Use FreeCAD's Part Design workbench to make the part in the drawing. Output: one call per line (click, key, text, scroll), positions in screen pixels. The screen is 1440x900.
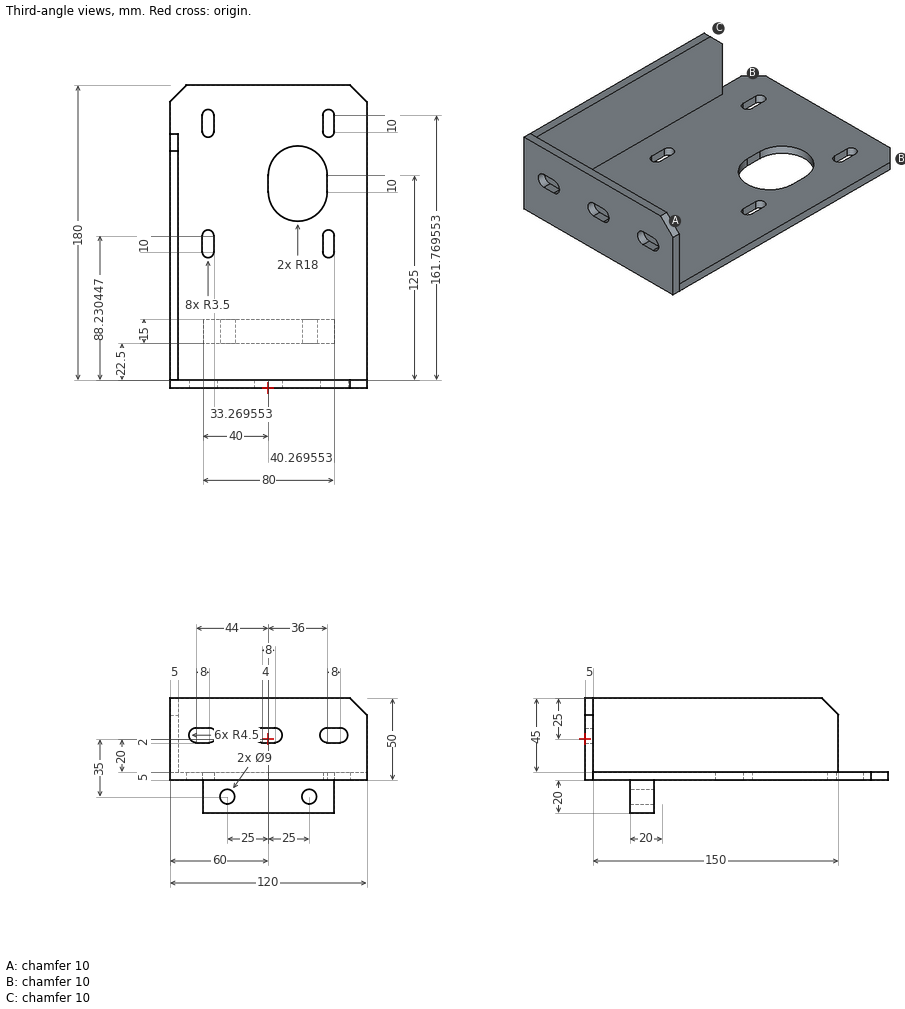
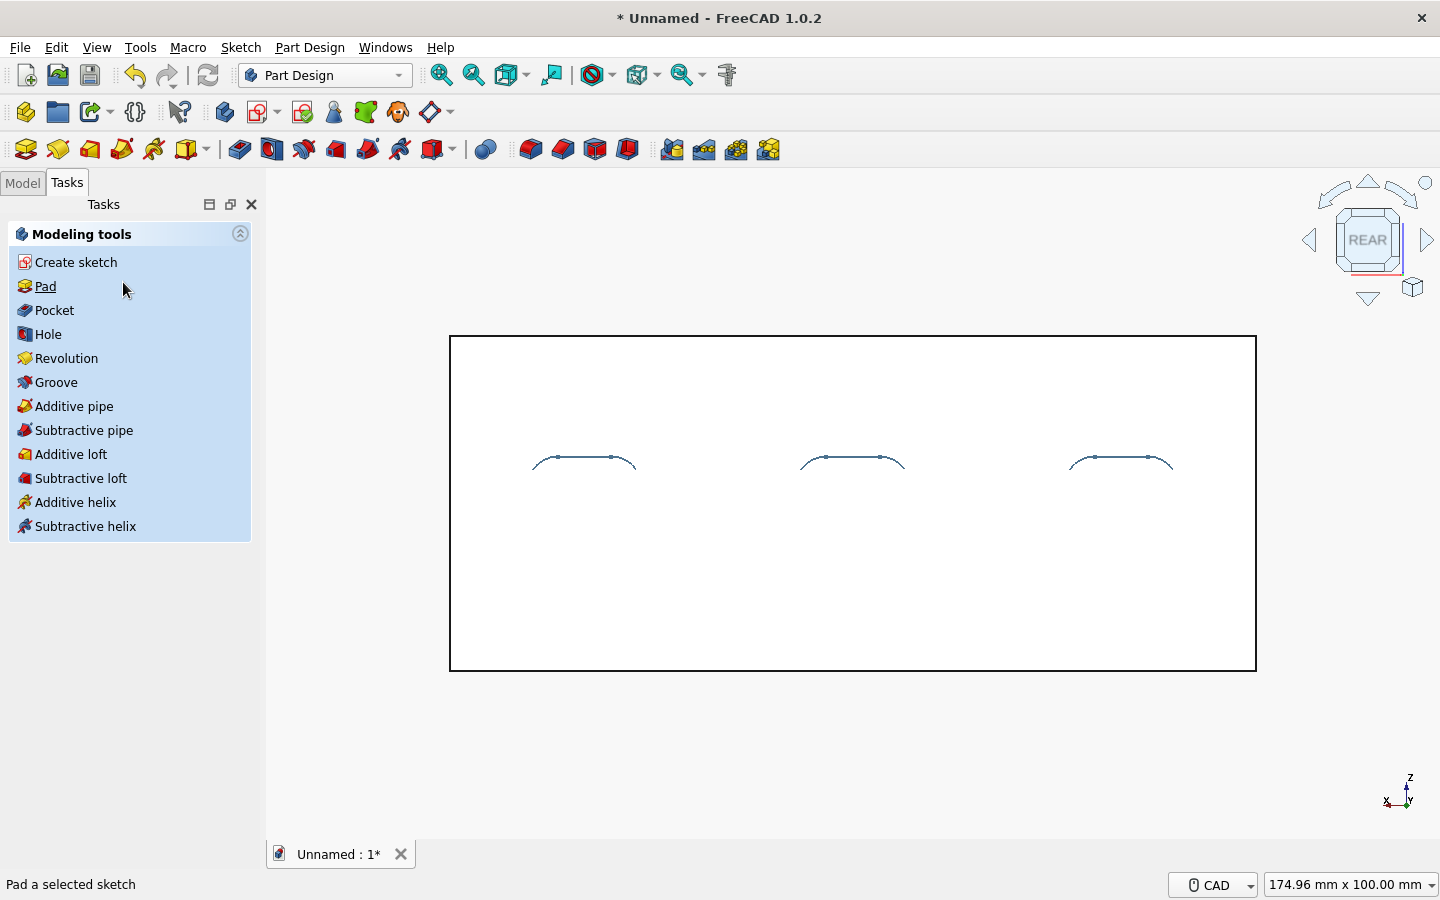
click(240, 150)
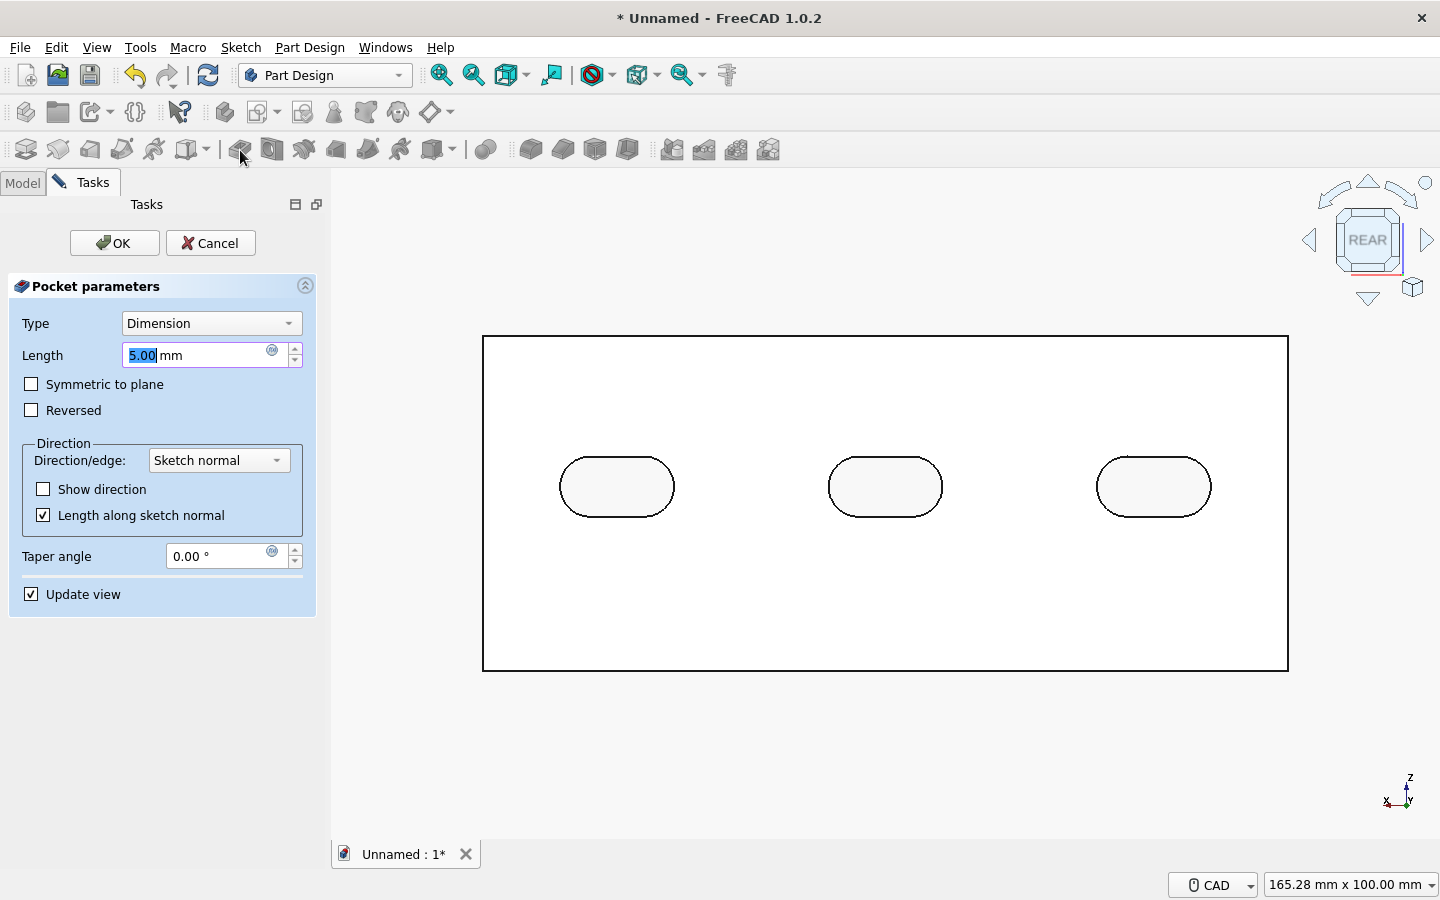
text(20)
key(Tab)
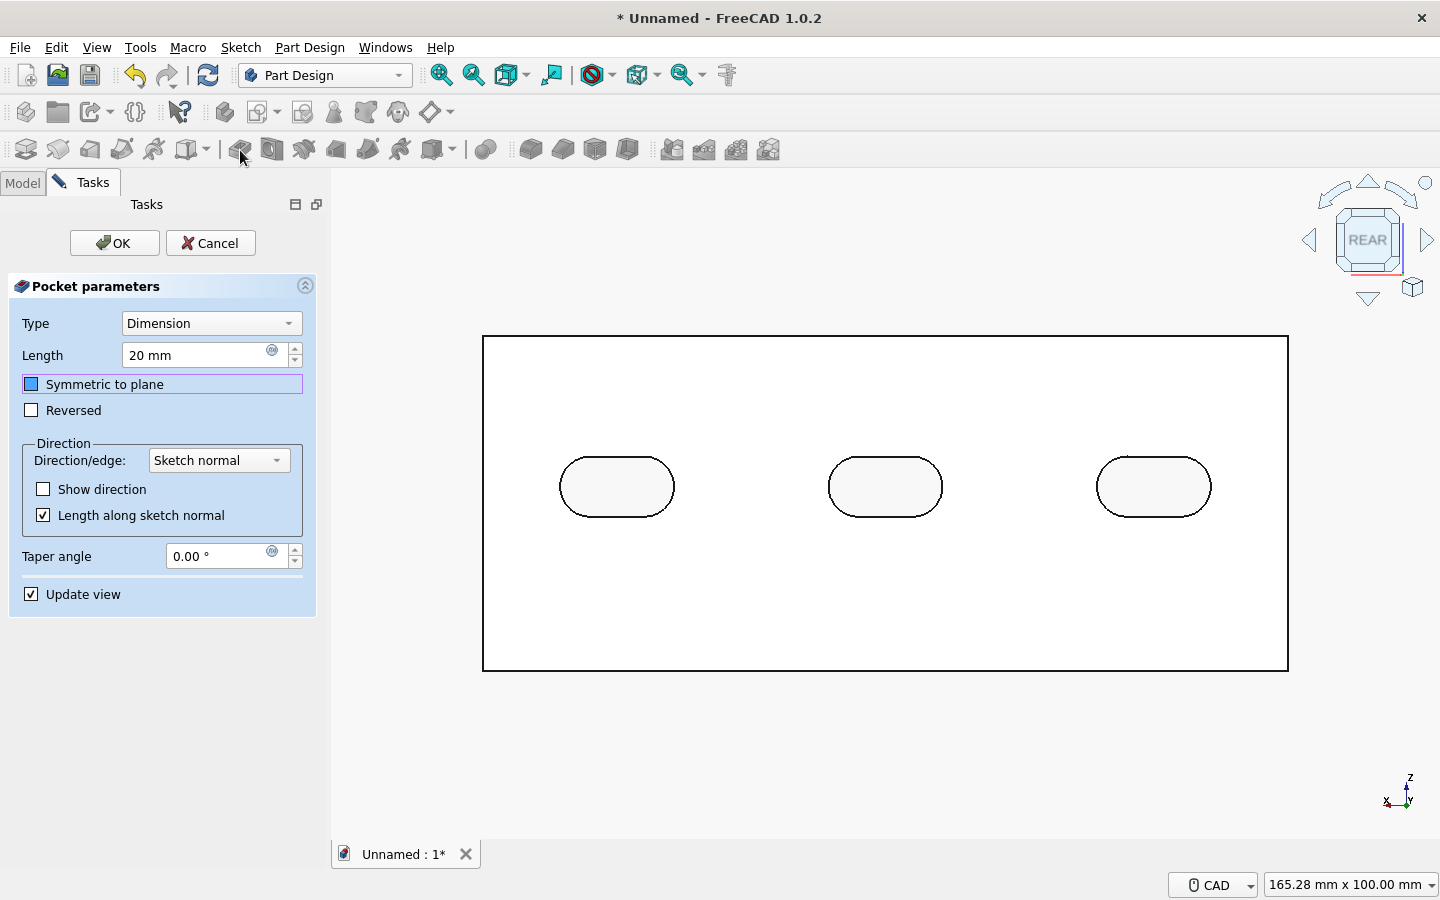
click(115, 243)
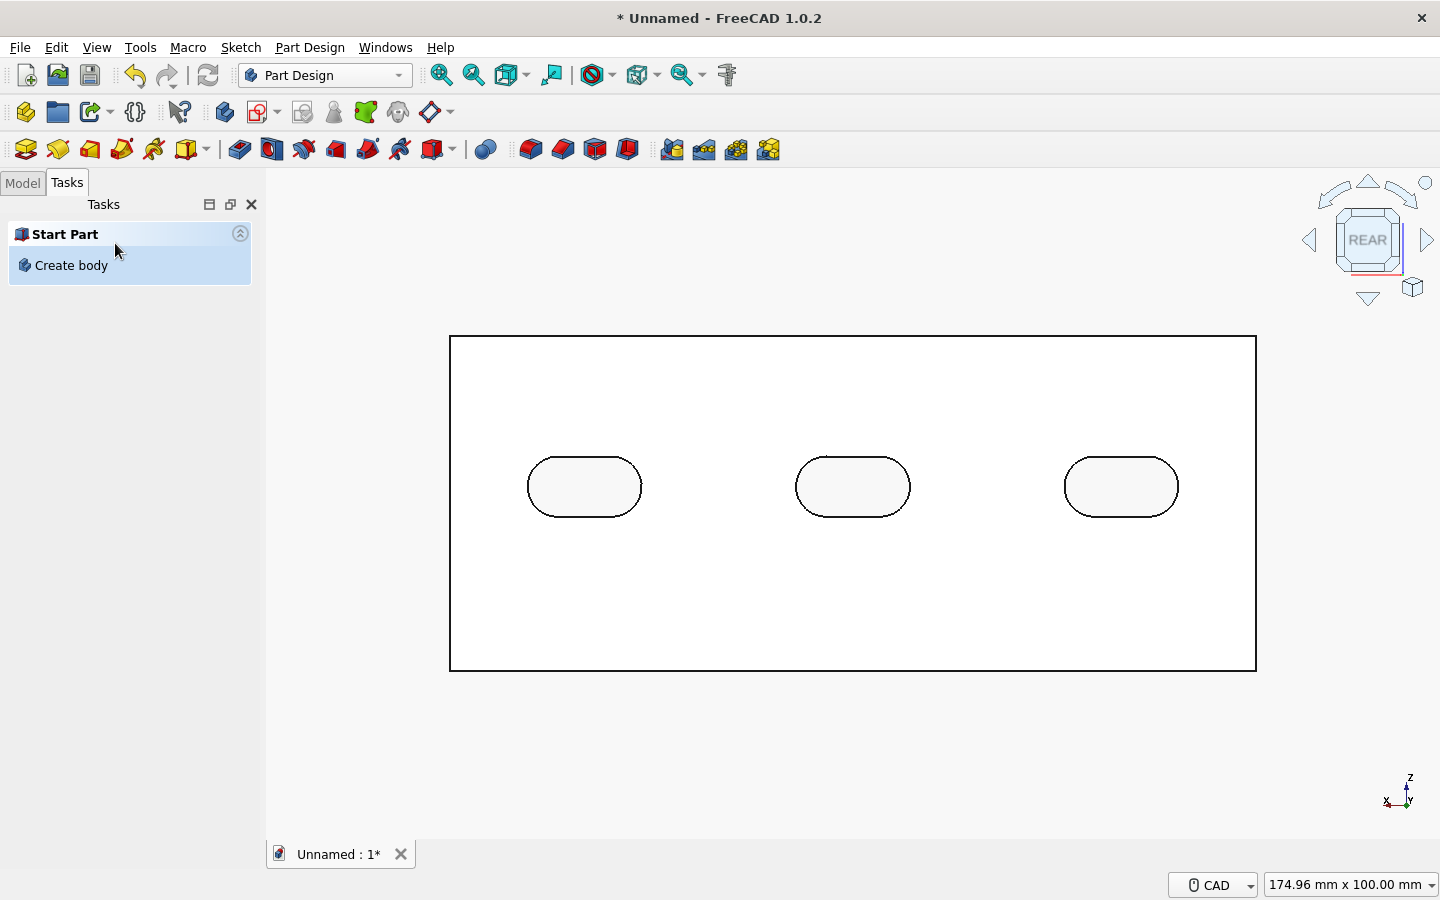
key(0)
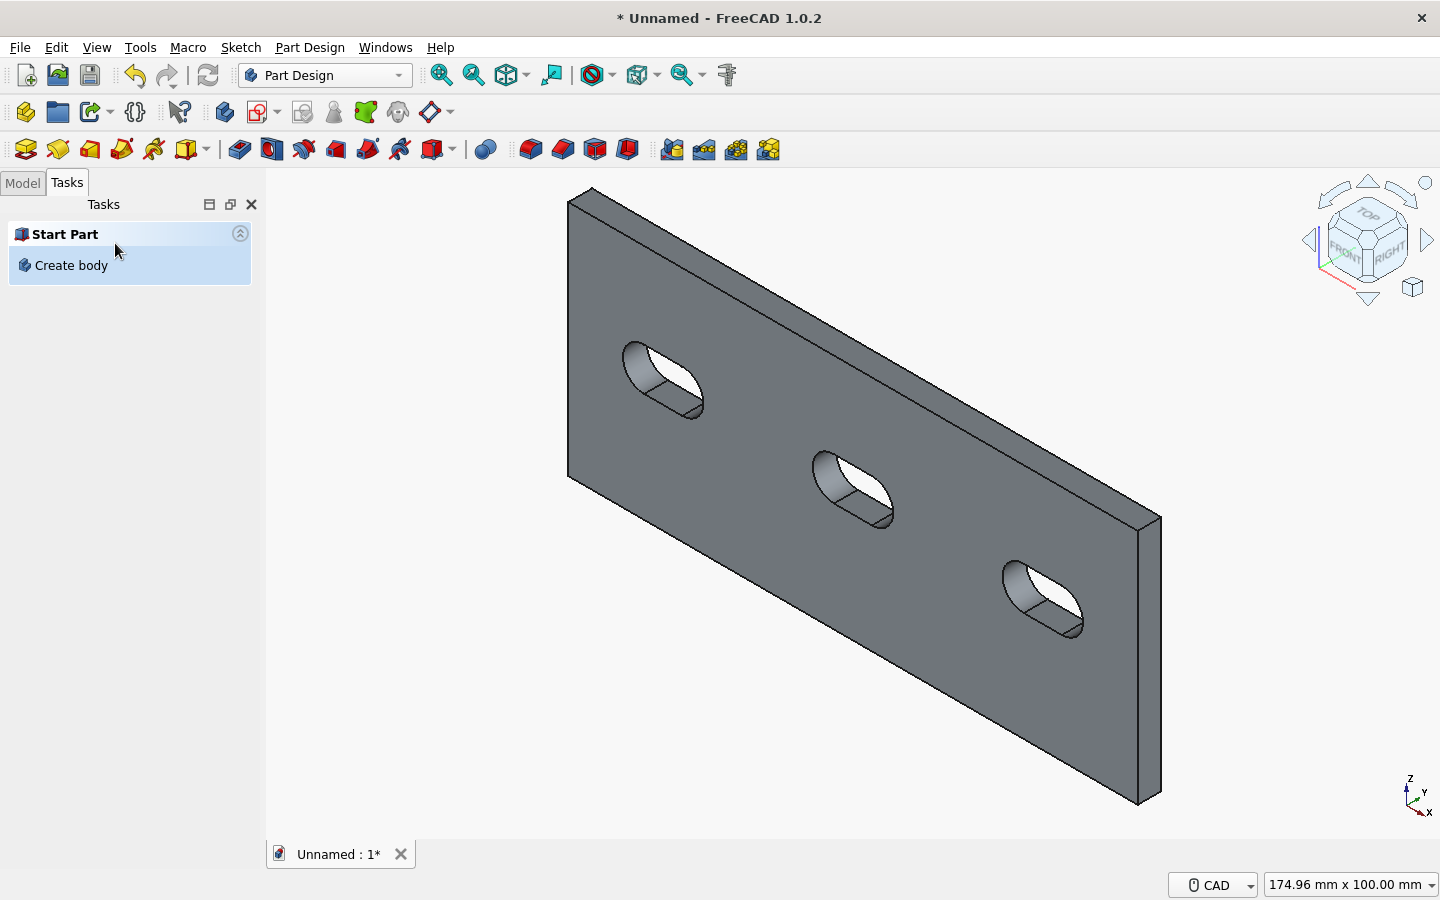
click(1150, 523)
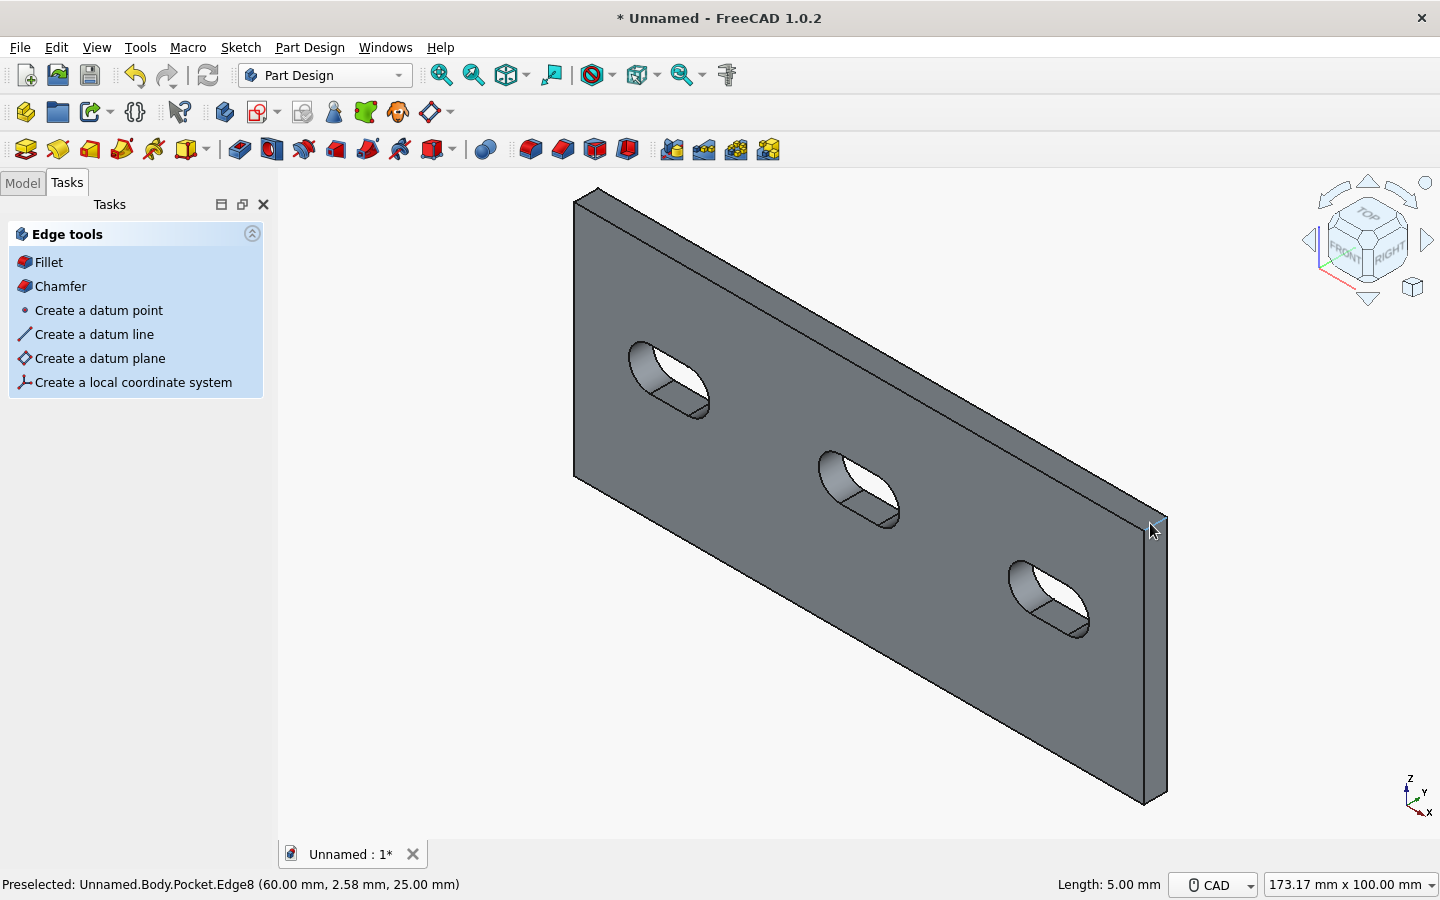
click(564, 150)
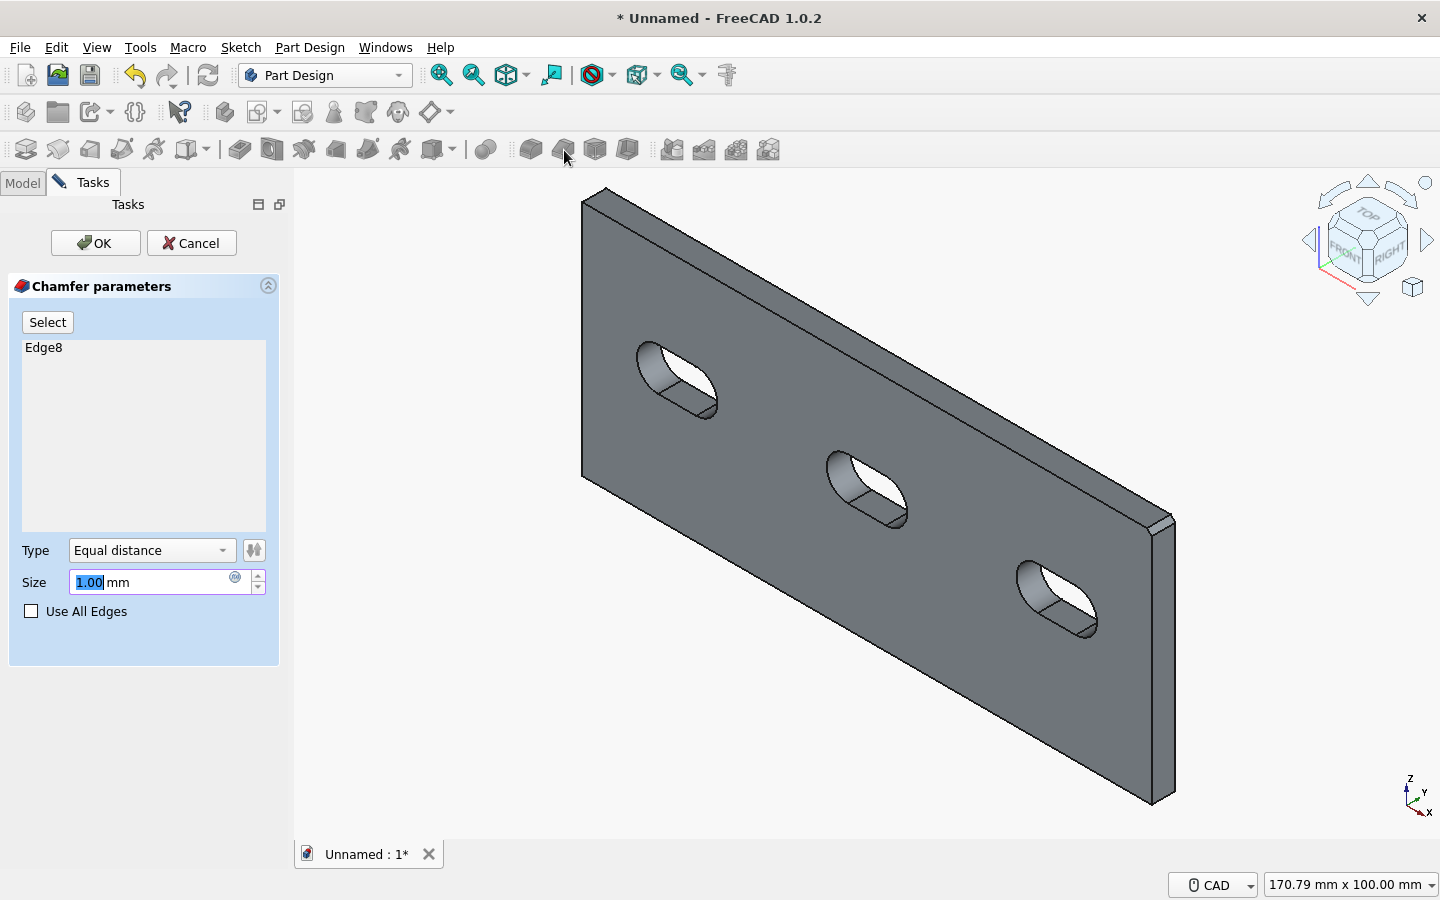
text(10)
key(Tab)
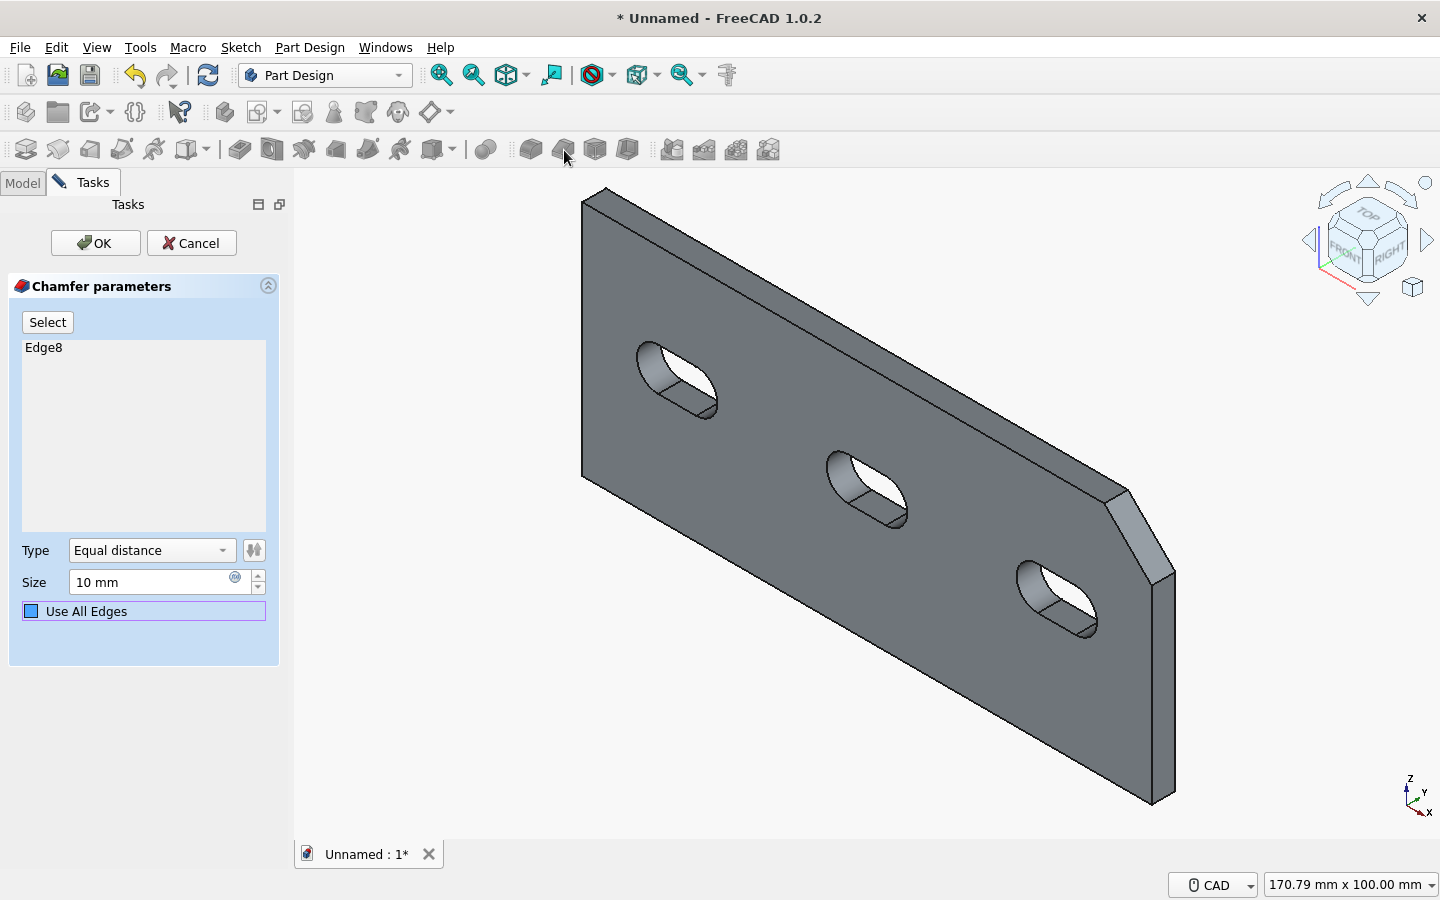
click(96, 243)